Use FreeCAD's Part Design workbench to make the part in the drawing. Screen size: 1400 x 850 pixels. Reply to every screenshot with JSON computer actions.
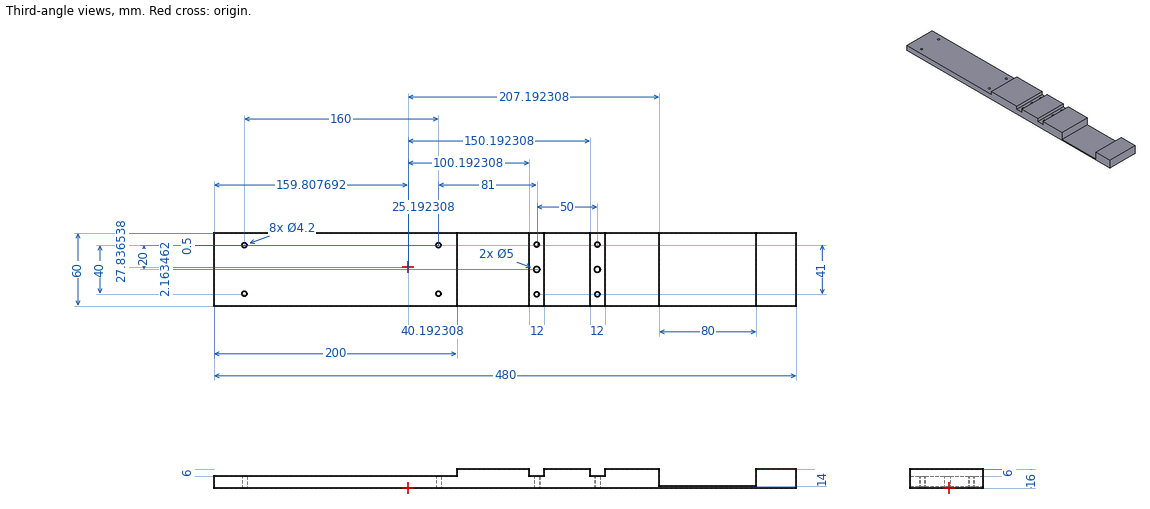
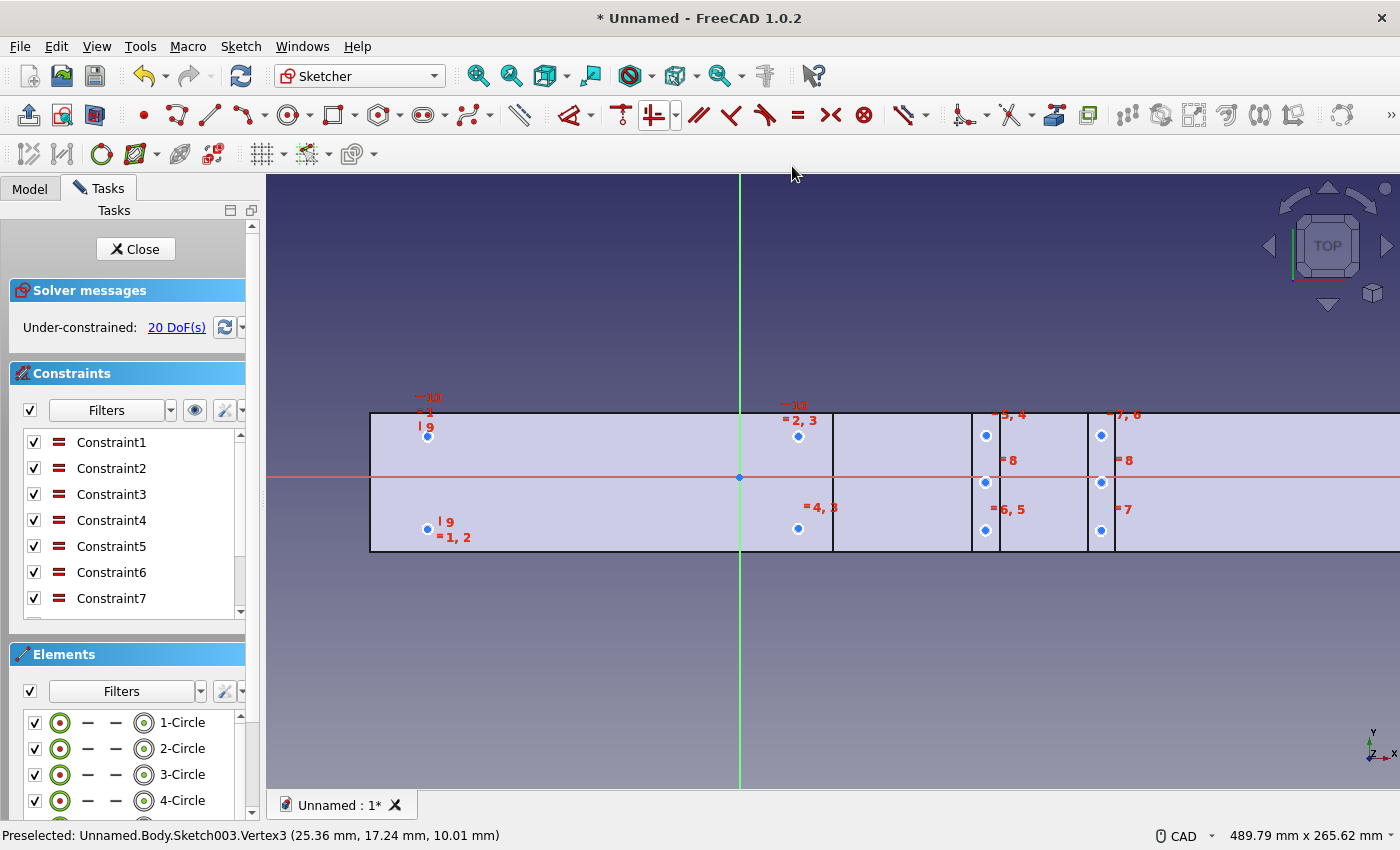
{"action": "left_click", "coordinate": [799, 437]}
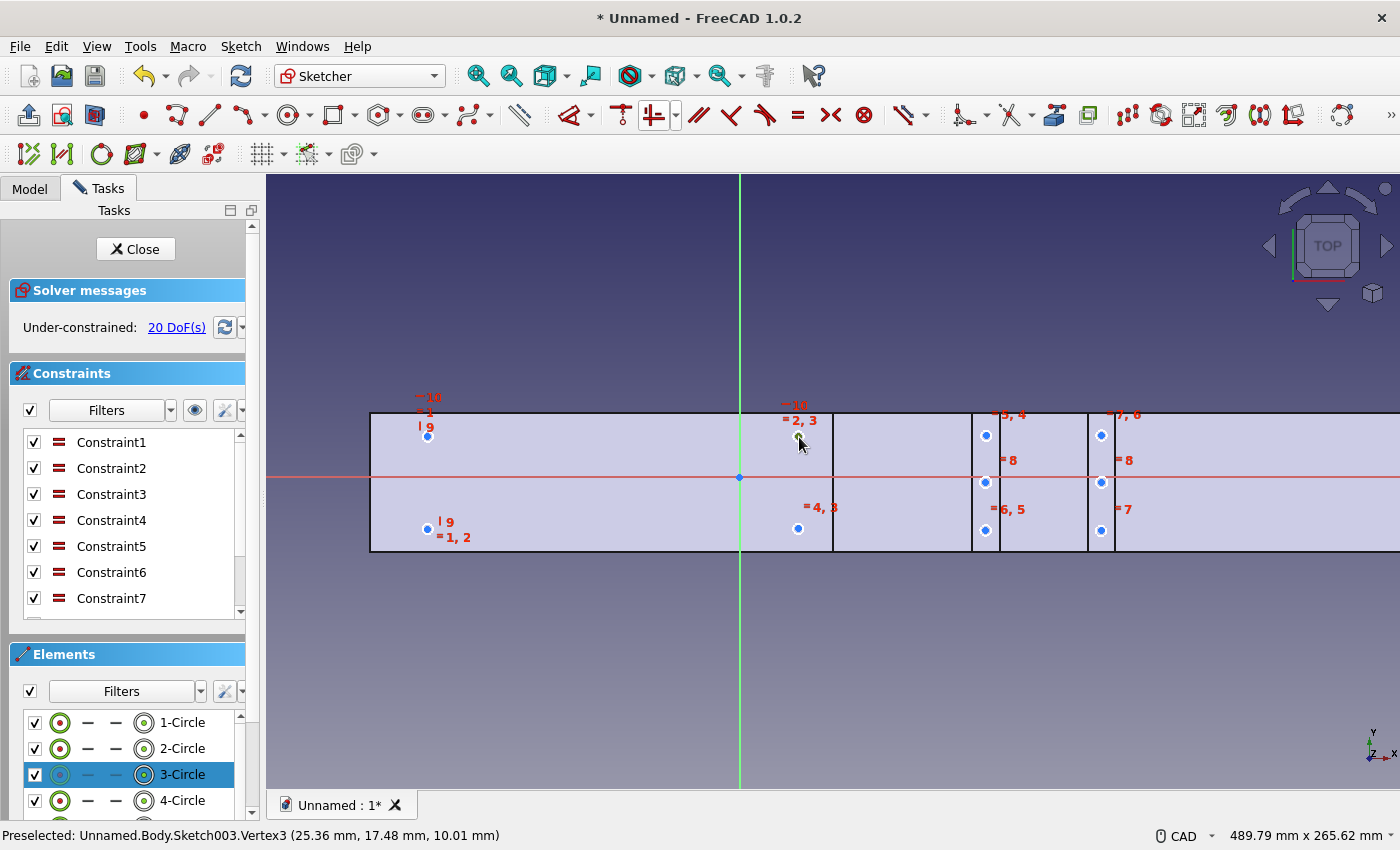
{"action": "left_click", "coordinate": [798, 529]}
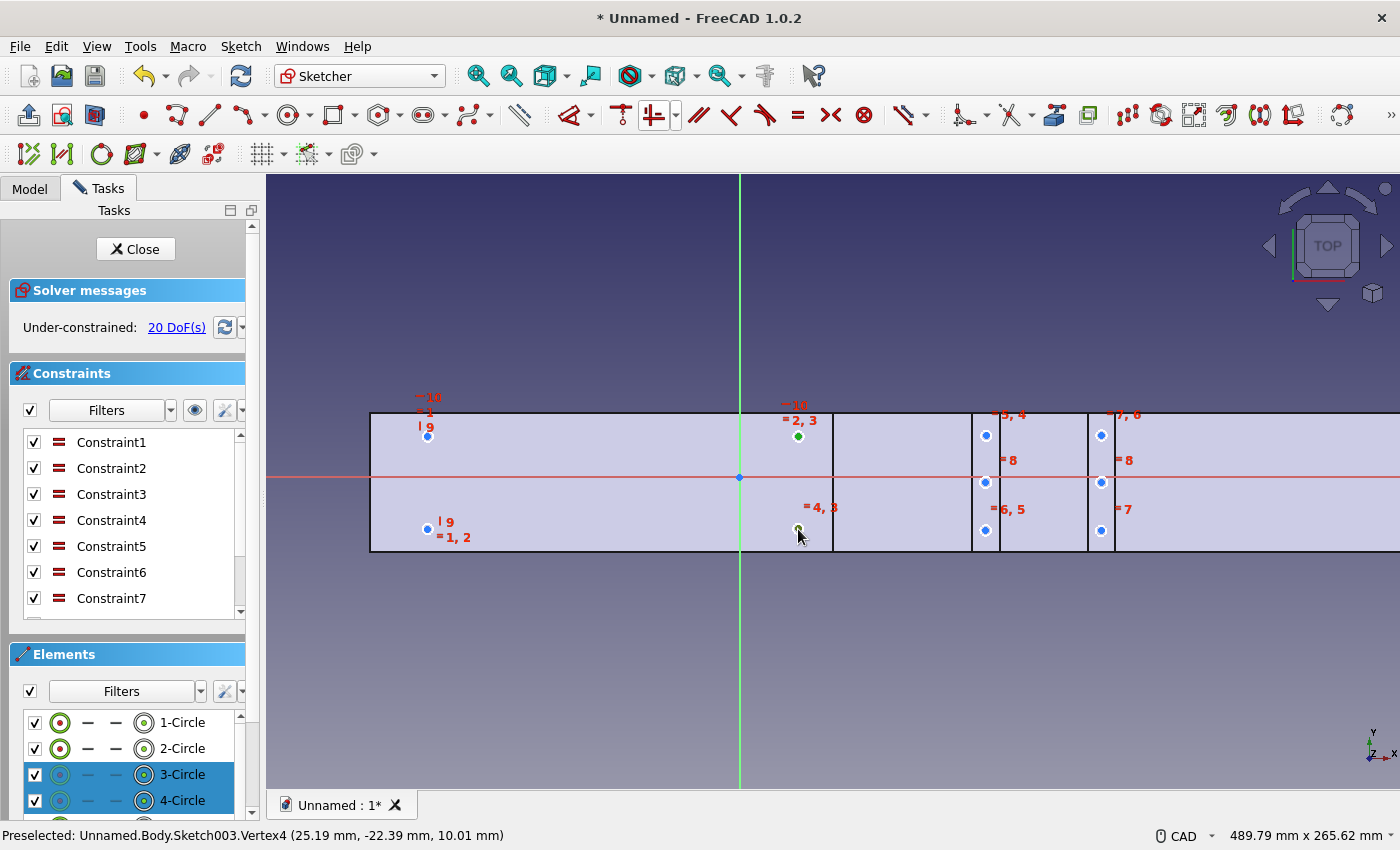
{"action": "key", "text": "v"}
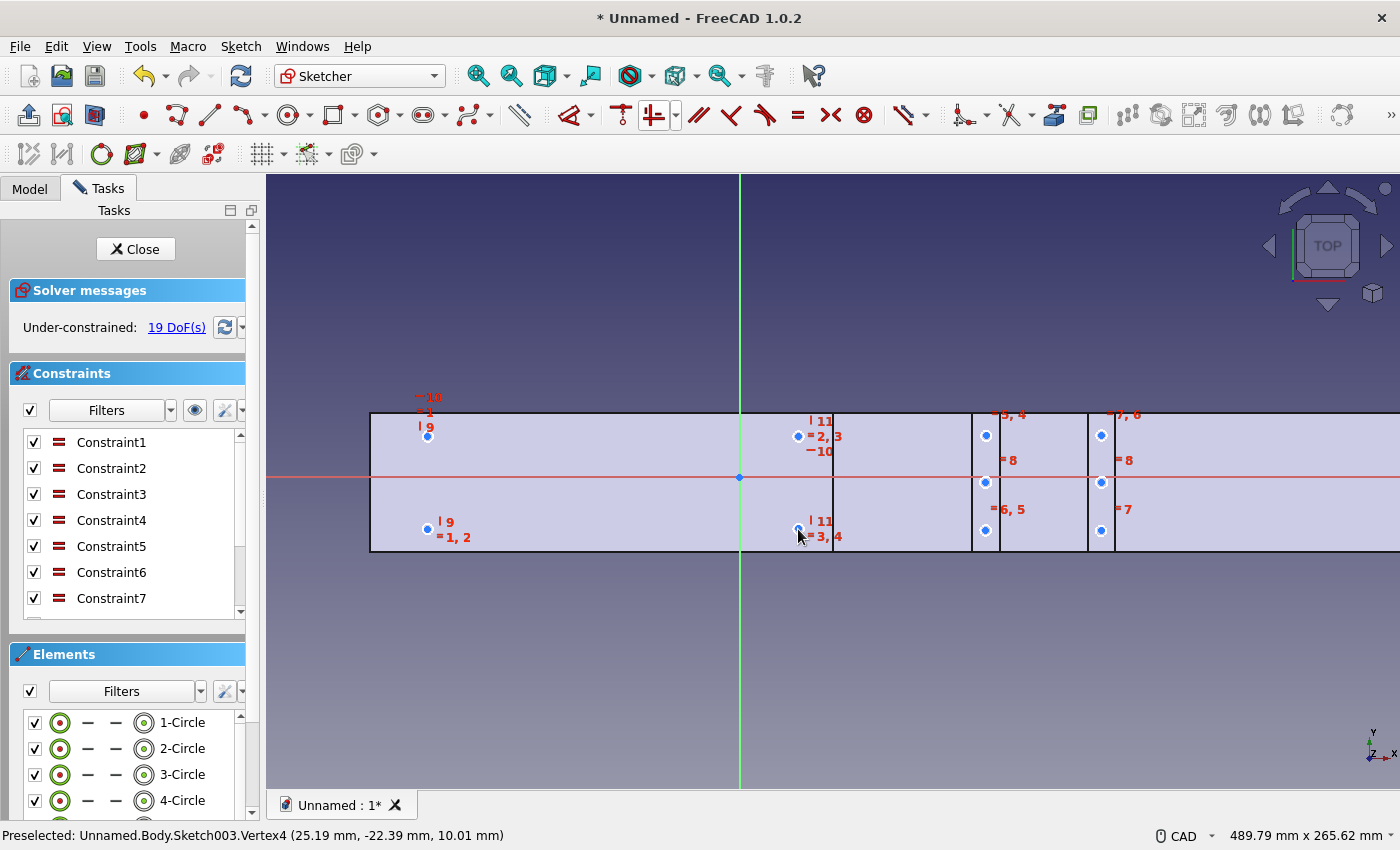
{"action": "left_click", "coordinate": [428, 529]}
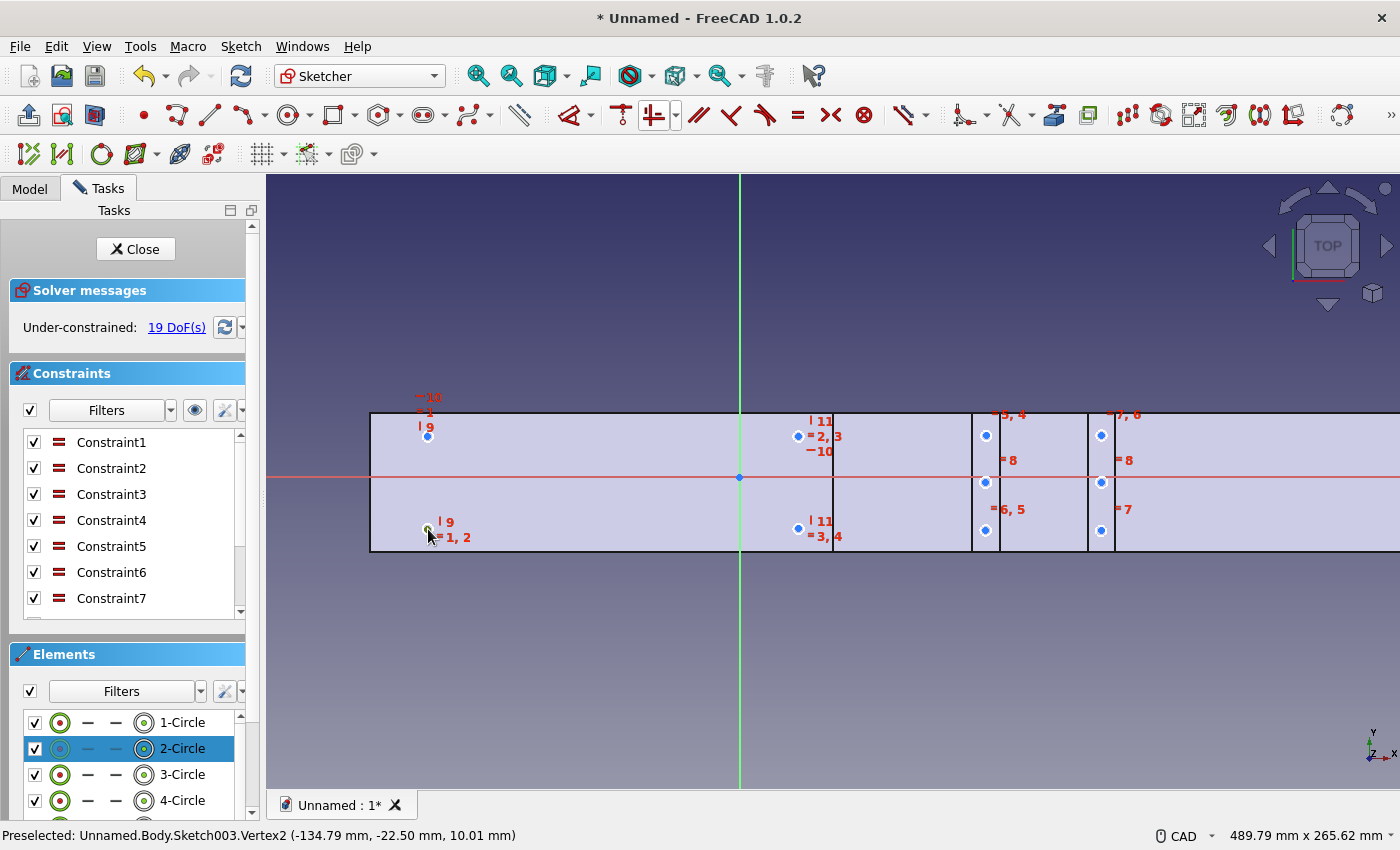
{"action": "left_click", "coordinate": [799, 529]}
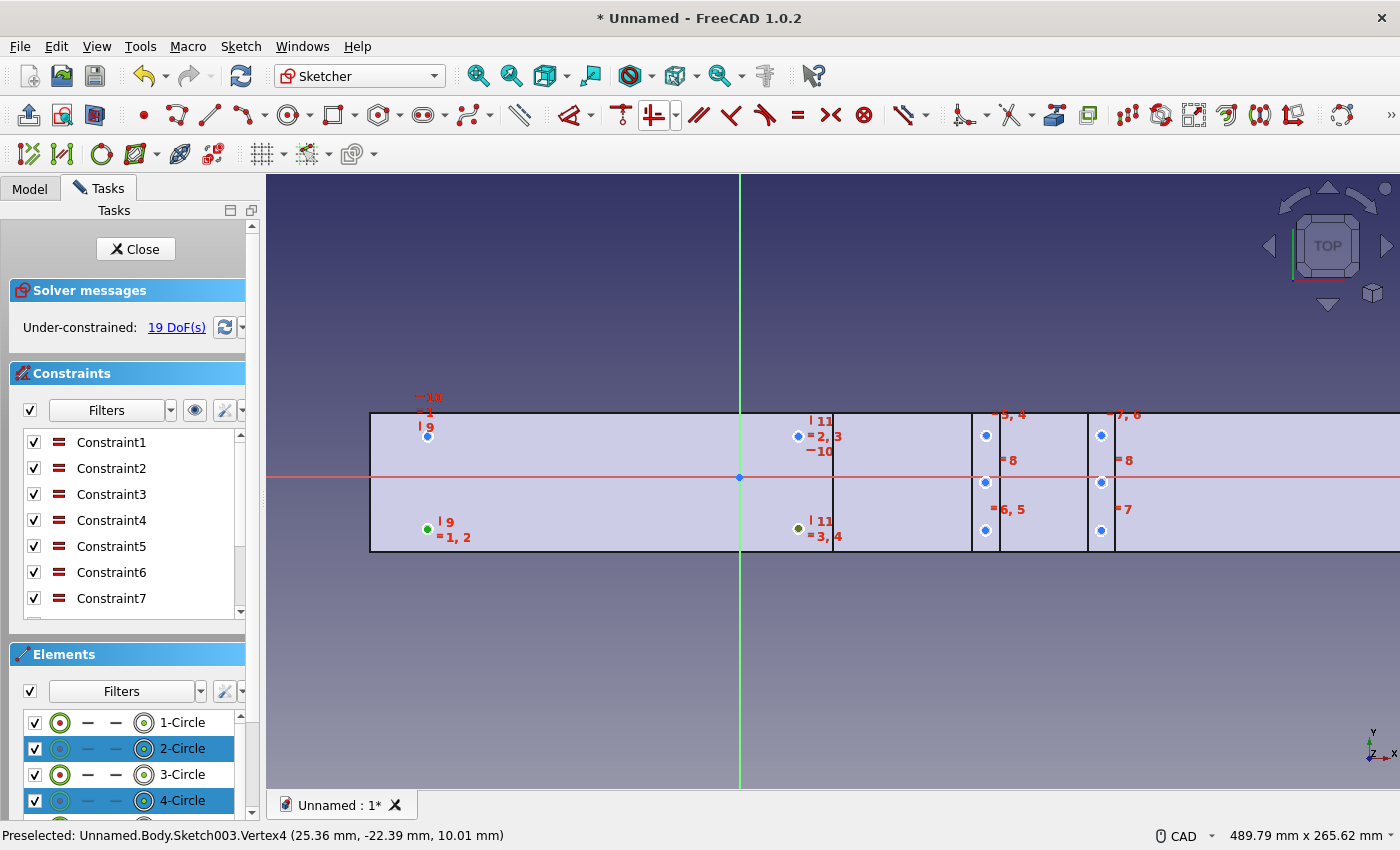
{"action": "key", "text": "h"}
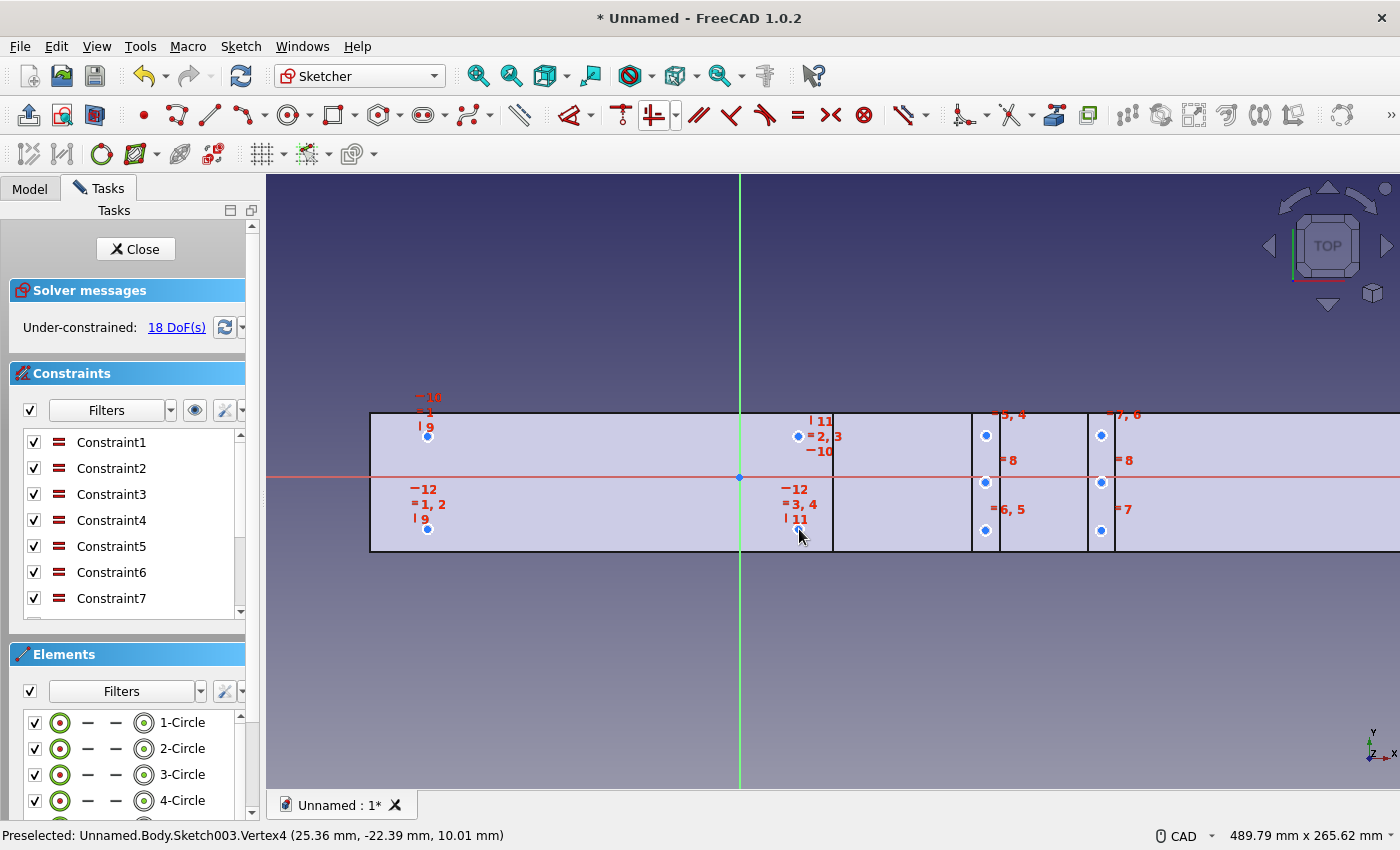
{"action": "left_click", "coordinate": [986, 436]}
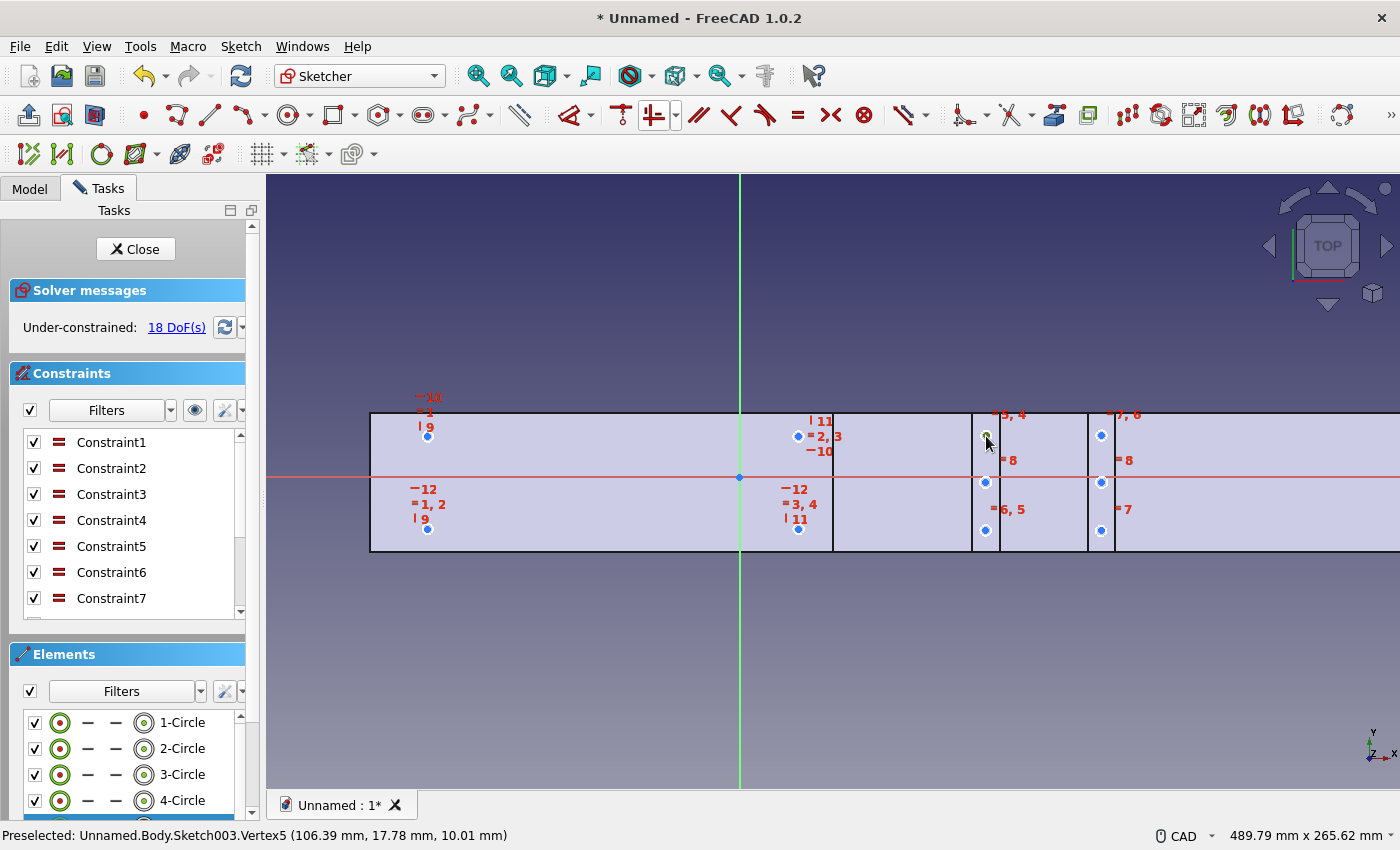
{"action": "left_click", "coordinate": [986, 530]}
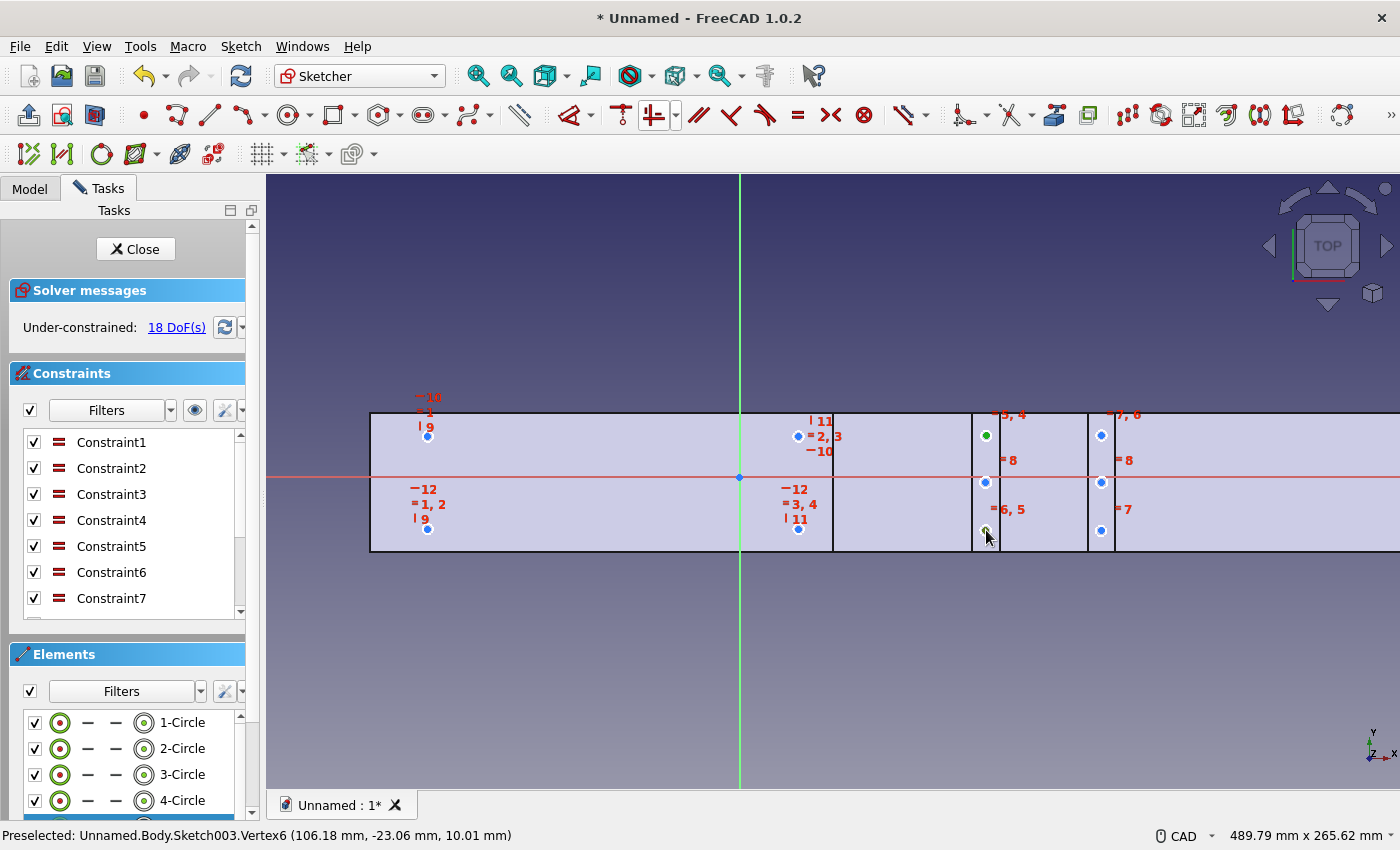
{"action": "key", "text": "v"}